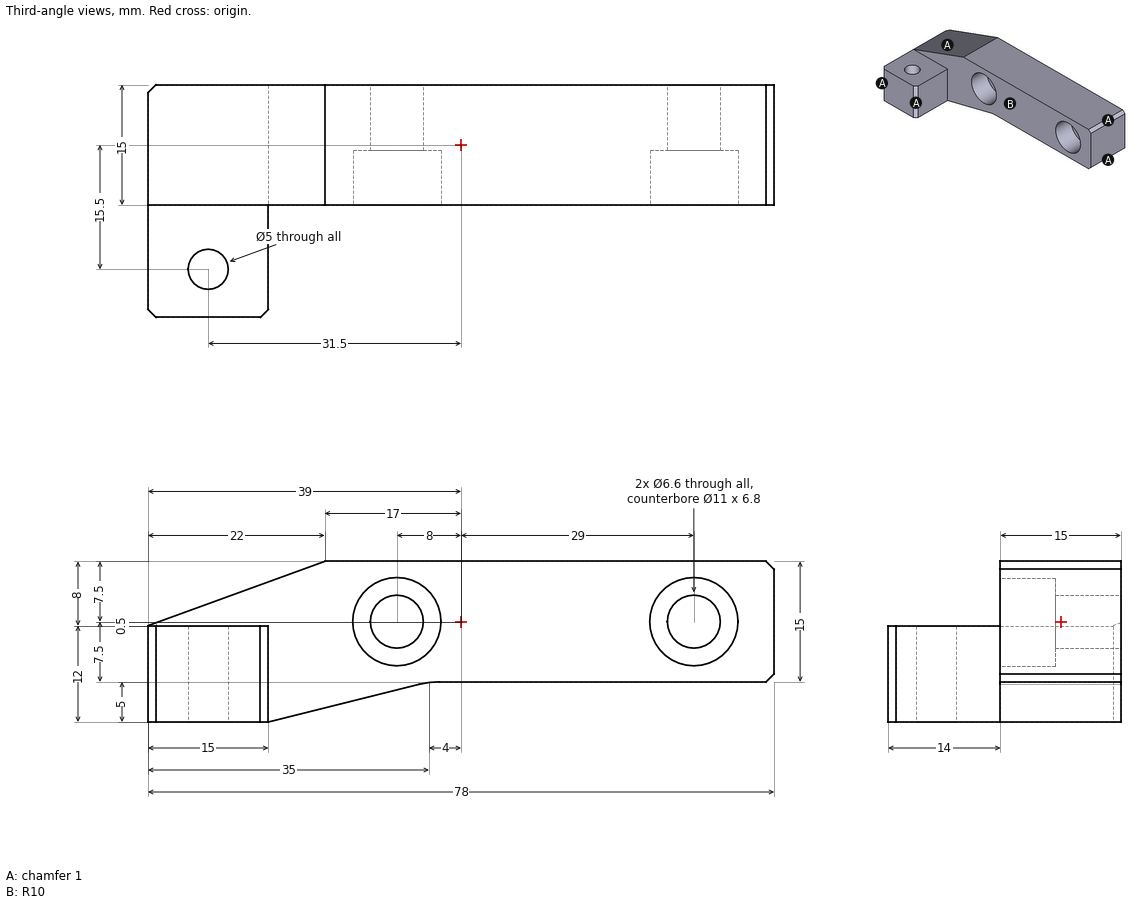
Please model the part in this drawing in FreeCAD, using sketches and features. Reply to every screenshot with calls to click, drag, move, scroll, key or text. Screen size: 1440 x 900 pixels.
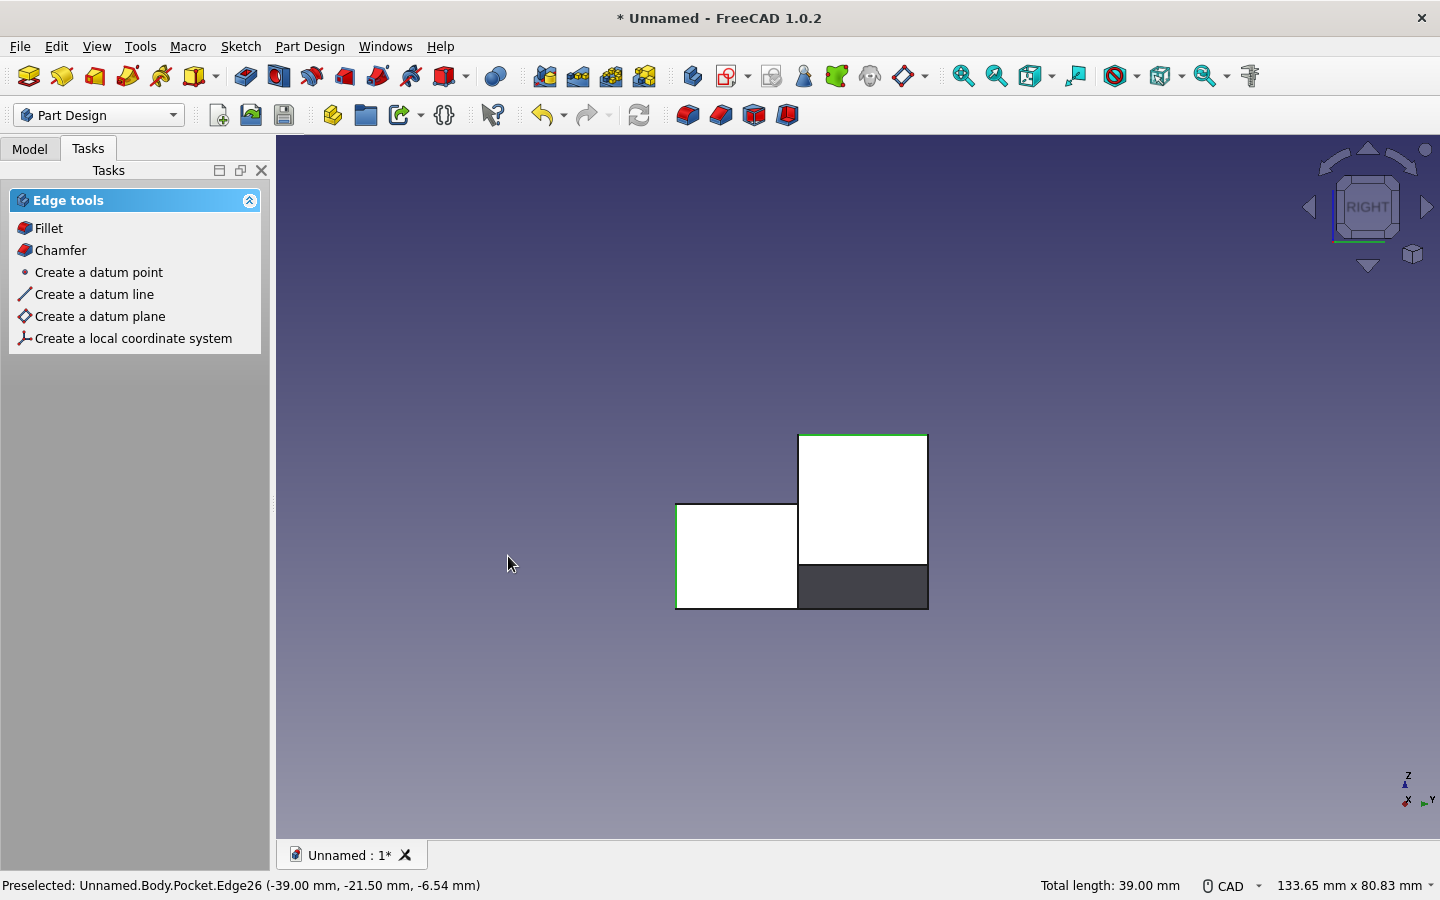
click(964, 76)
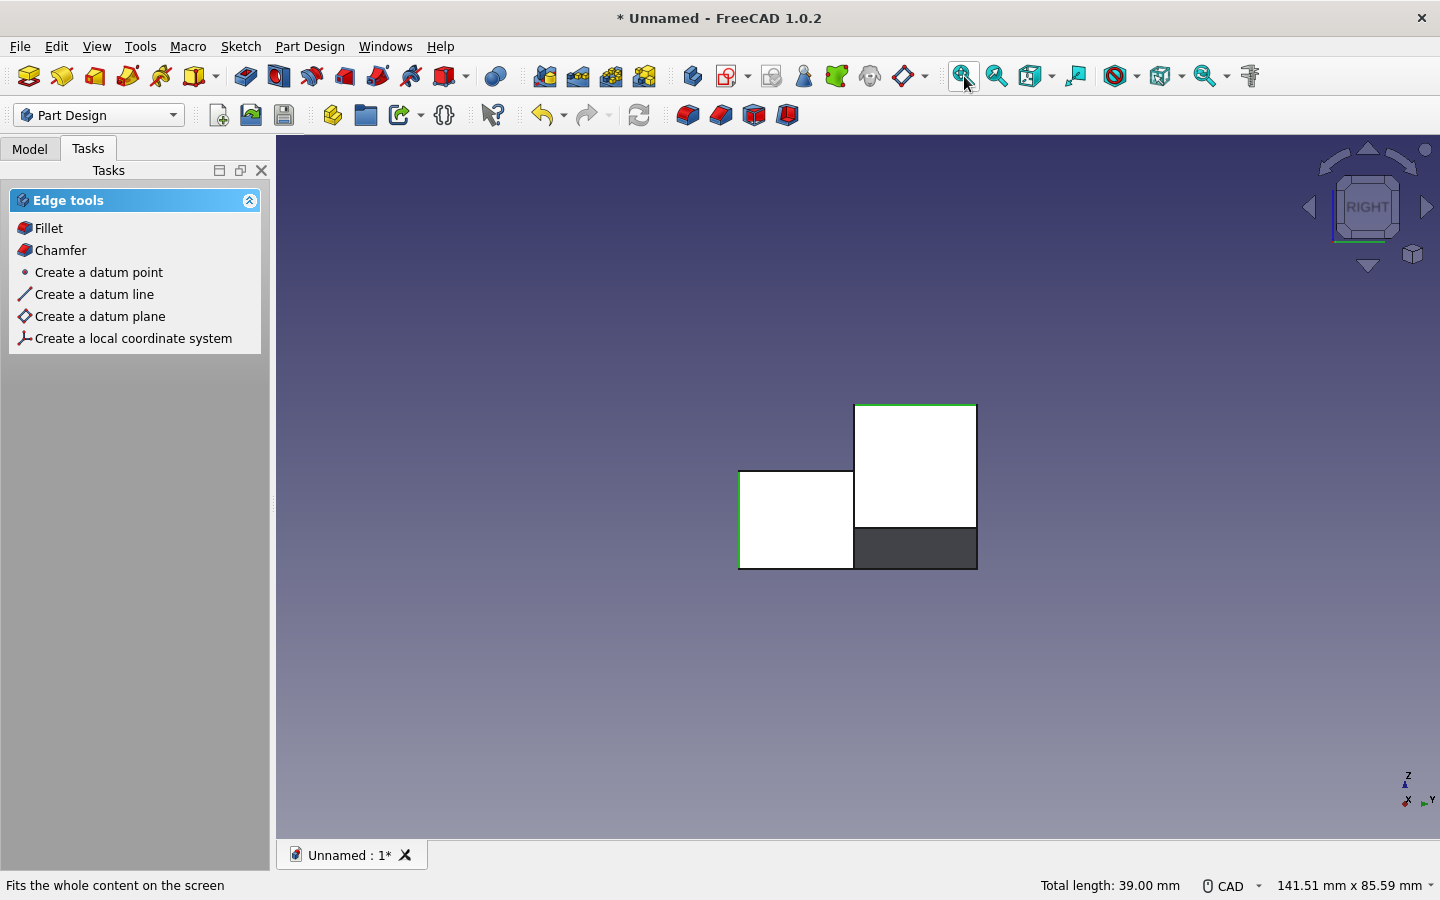
click(916, 527, ctrl)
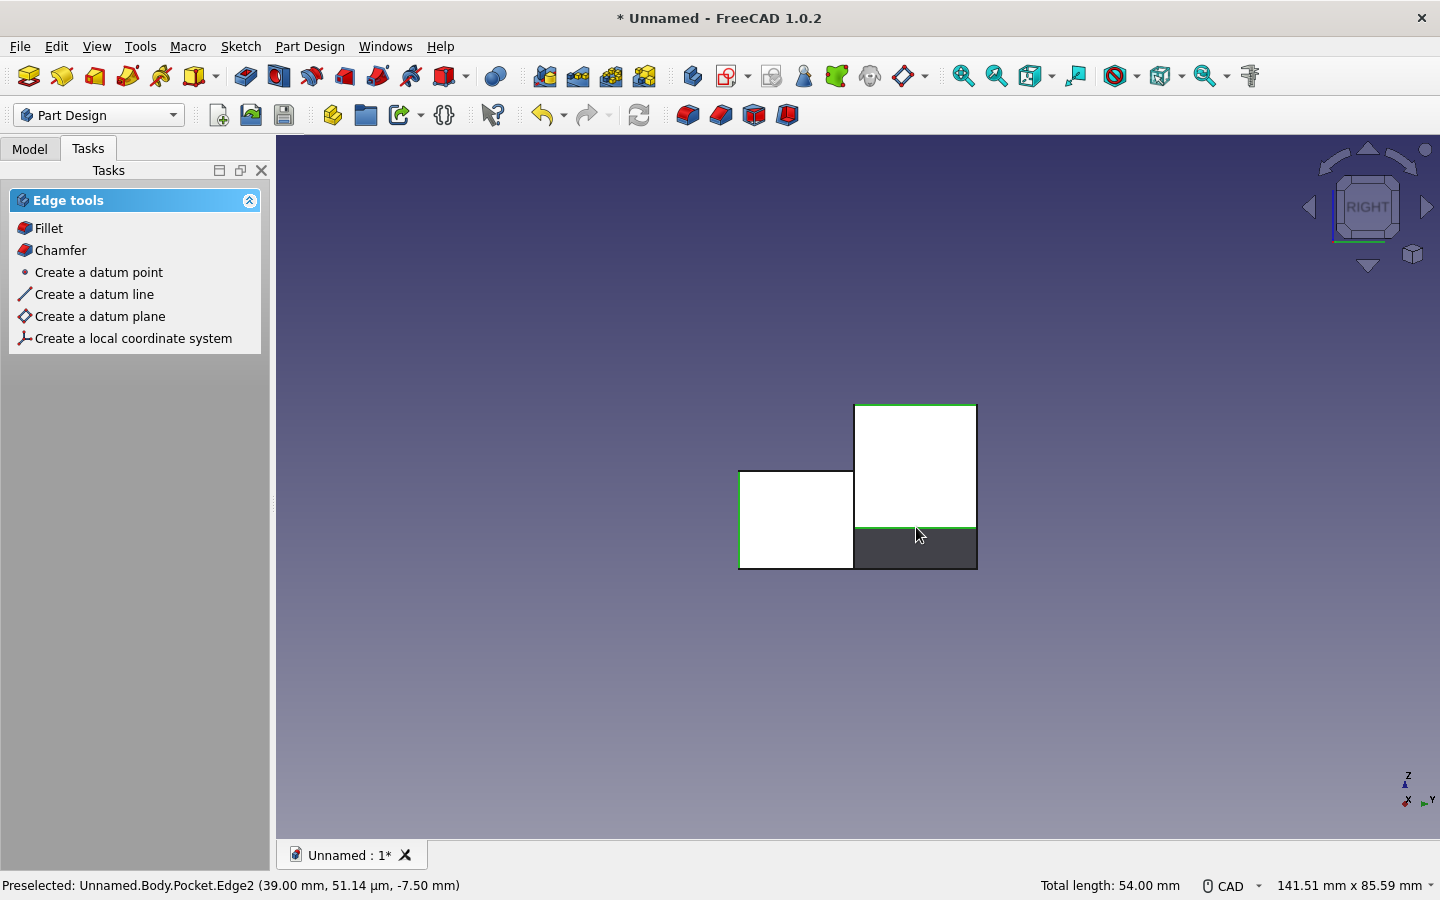
key(5)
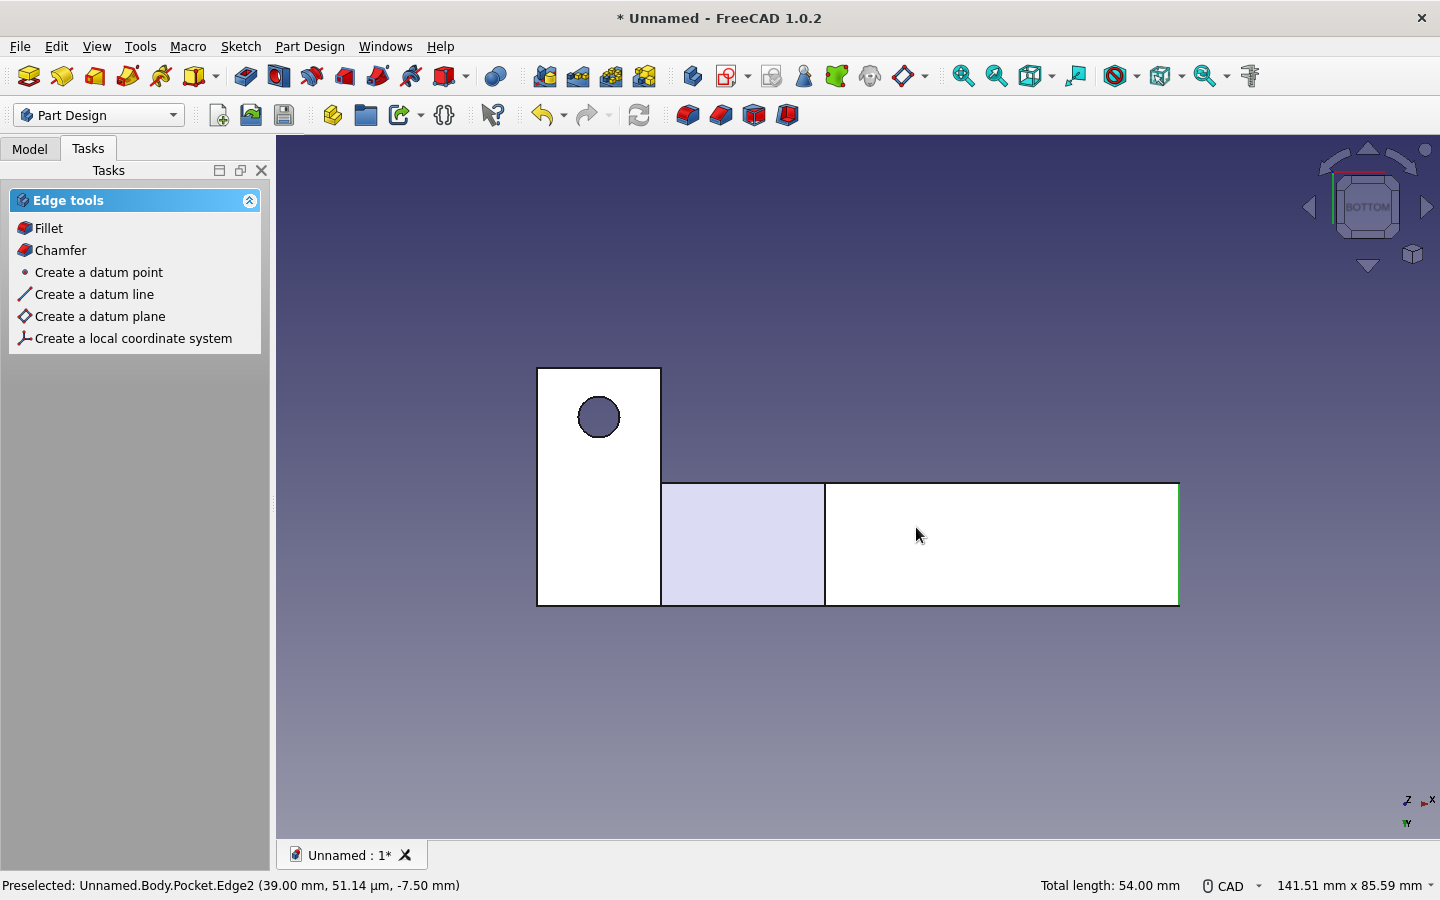
key(4)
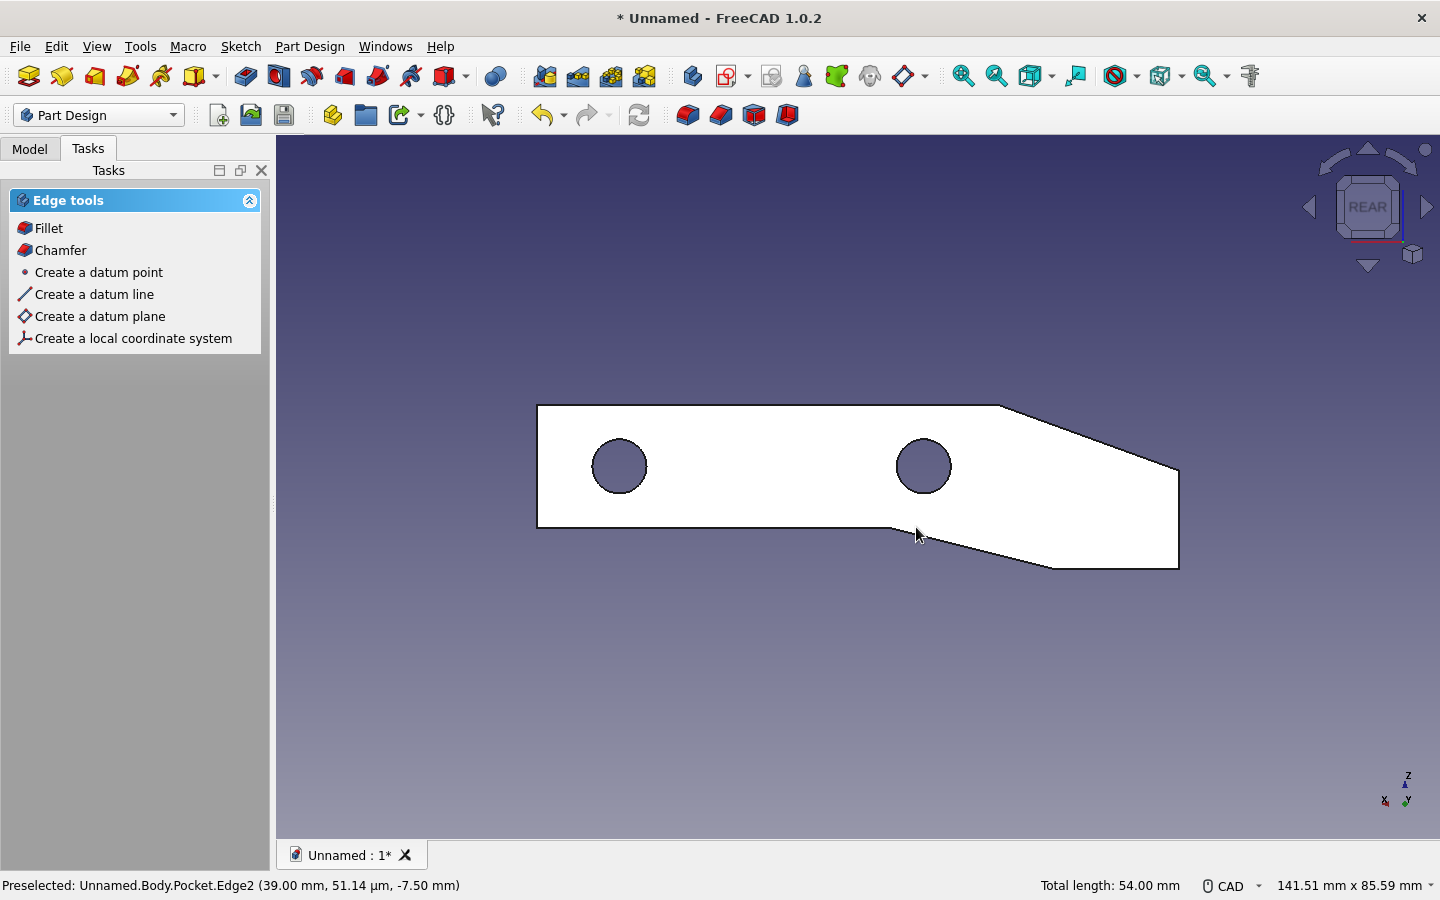
click(1179, 519, ctrl)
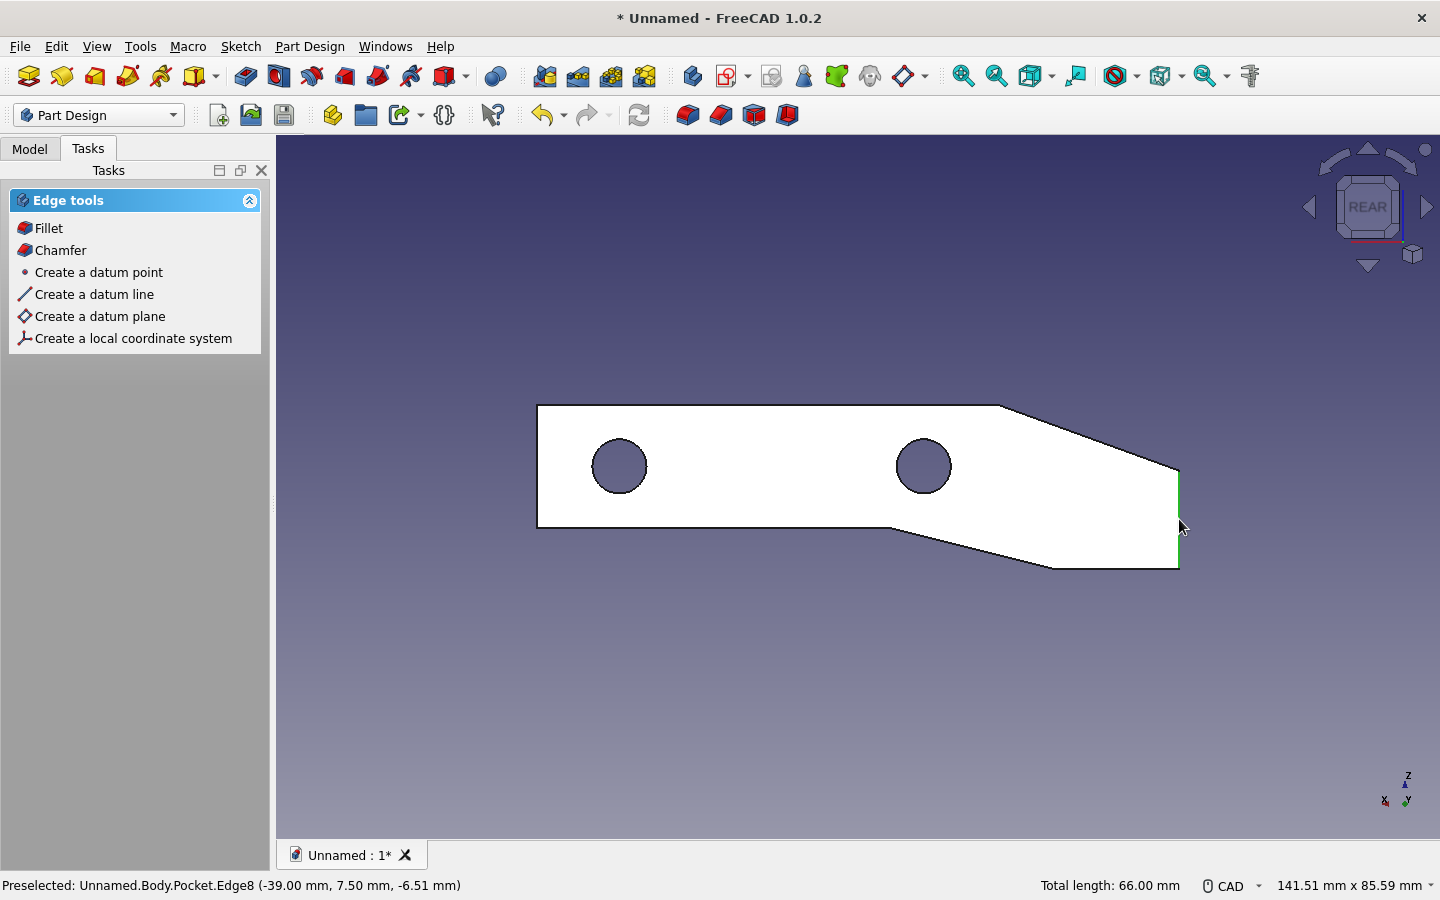
click(721, 116)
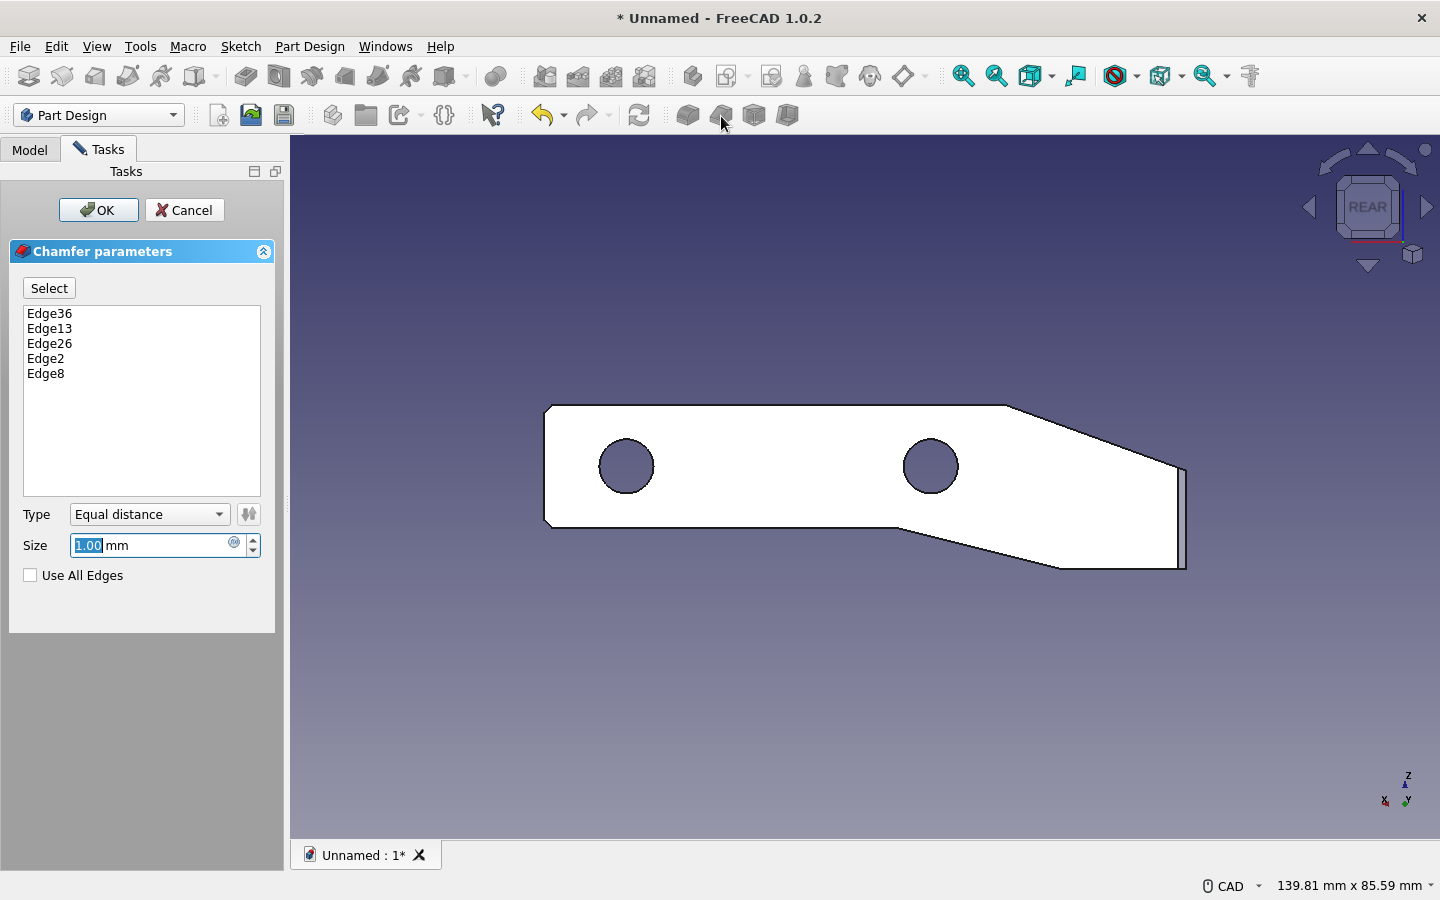
text(1)
key(Tab)